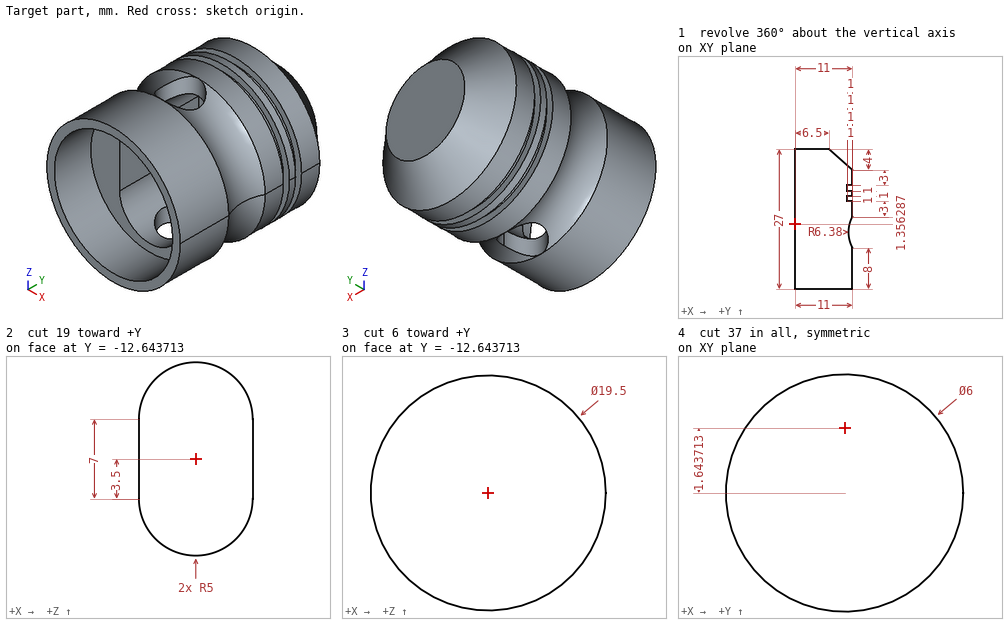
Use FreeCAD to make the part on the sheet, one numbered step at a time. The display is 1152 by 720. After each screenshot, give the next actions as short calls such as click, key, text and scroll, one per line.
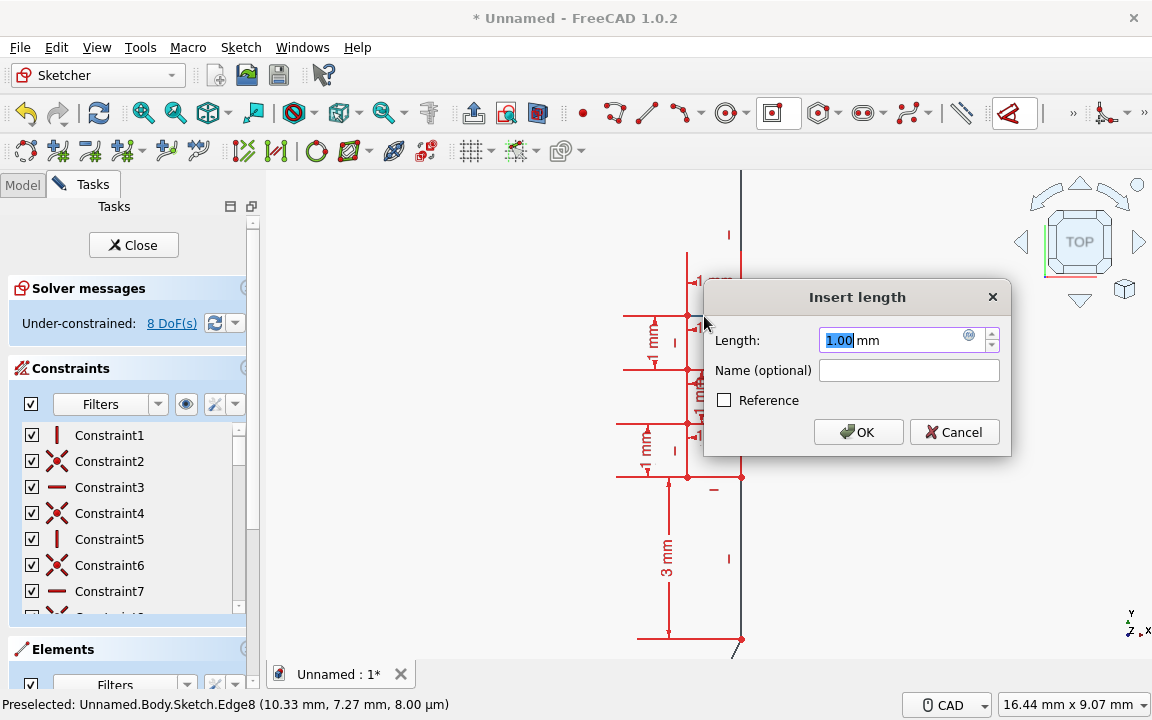
text(1)
key(Return)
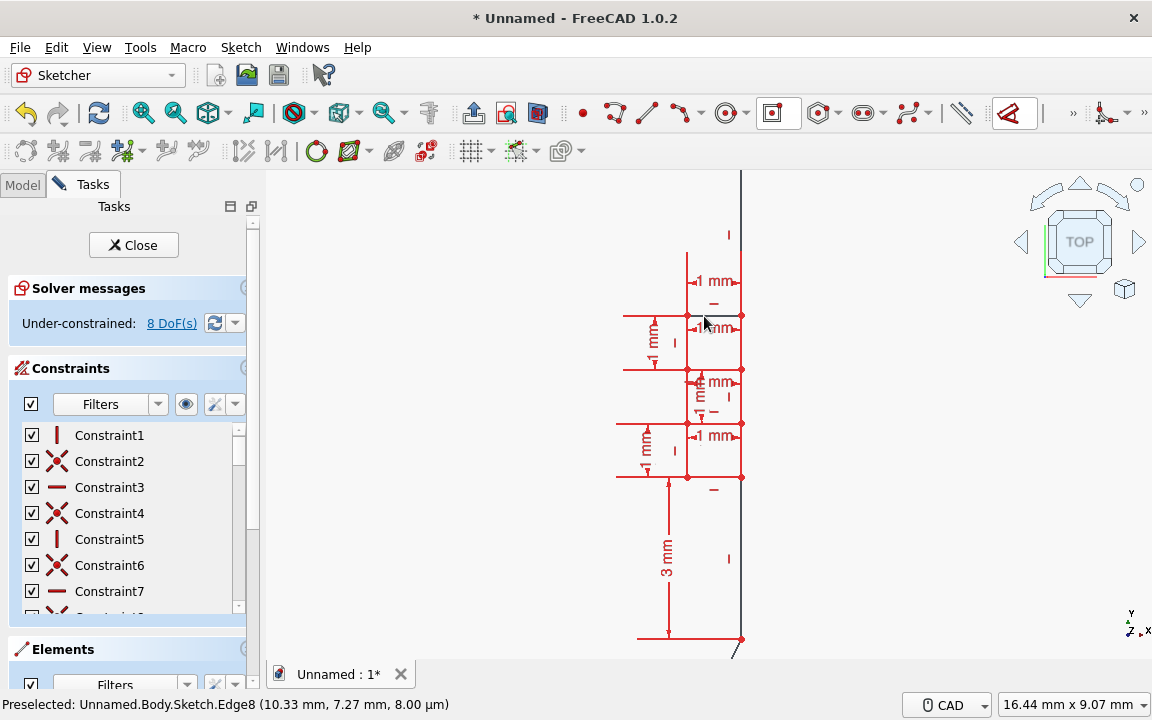
scroll(690, 352, down, 8)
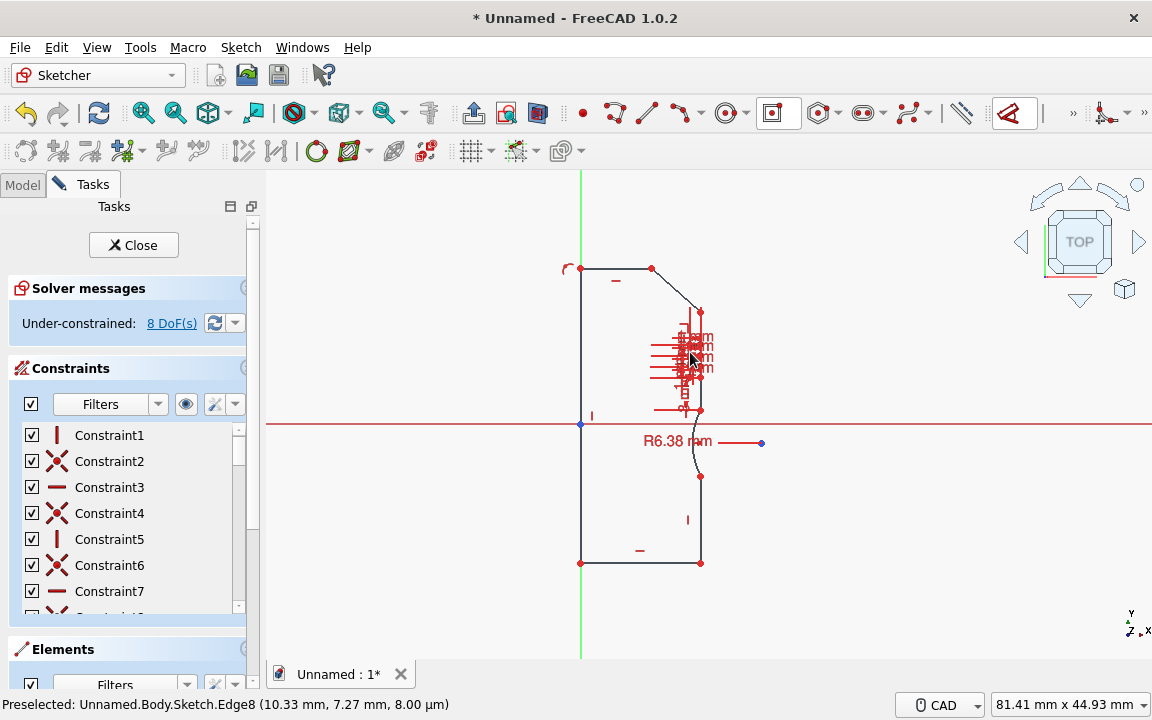
scroll(701, 335, up, 2)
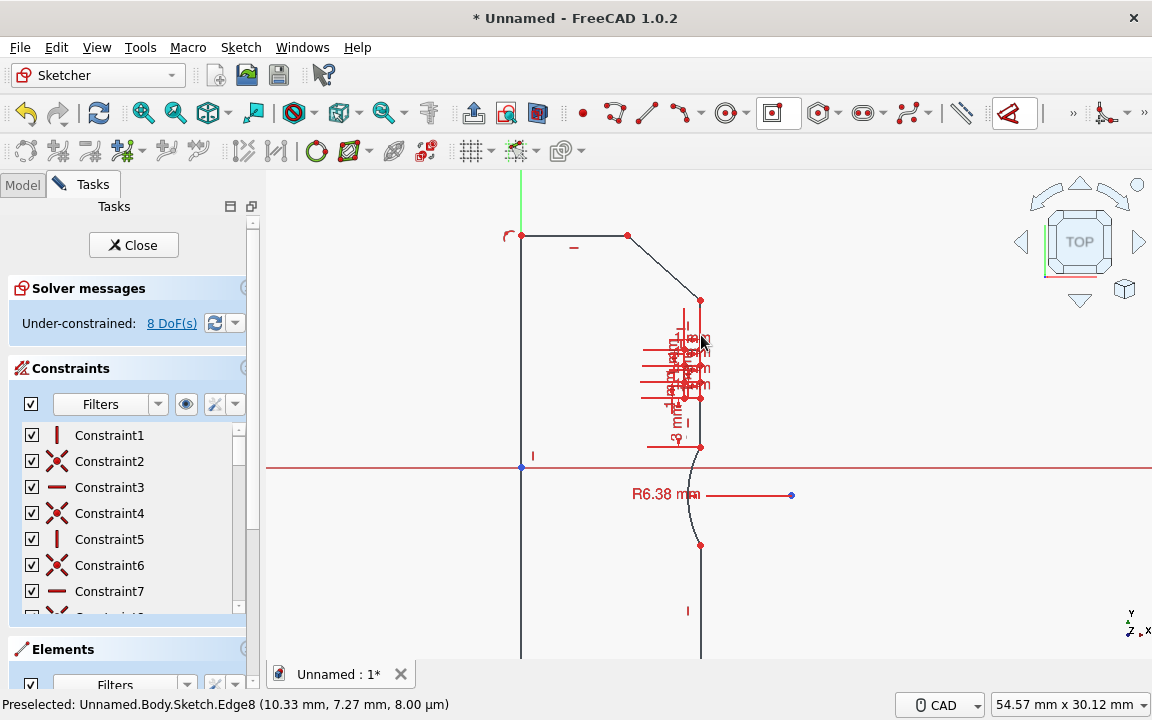
click(700, 315)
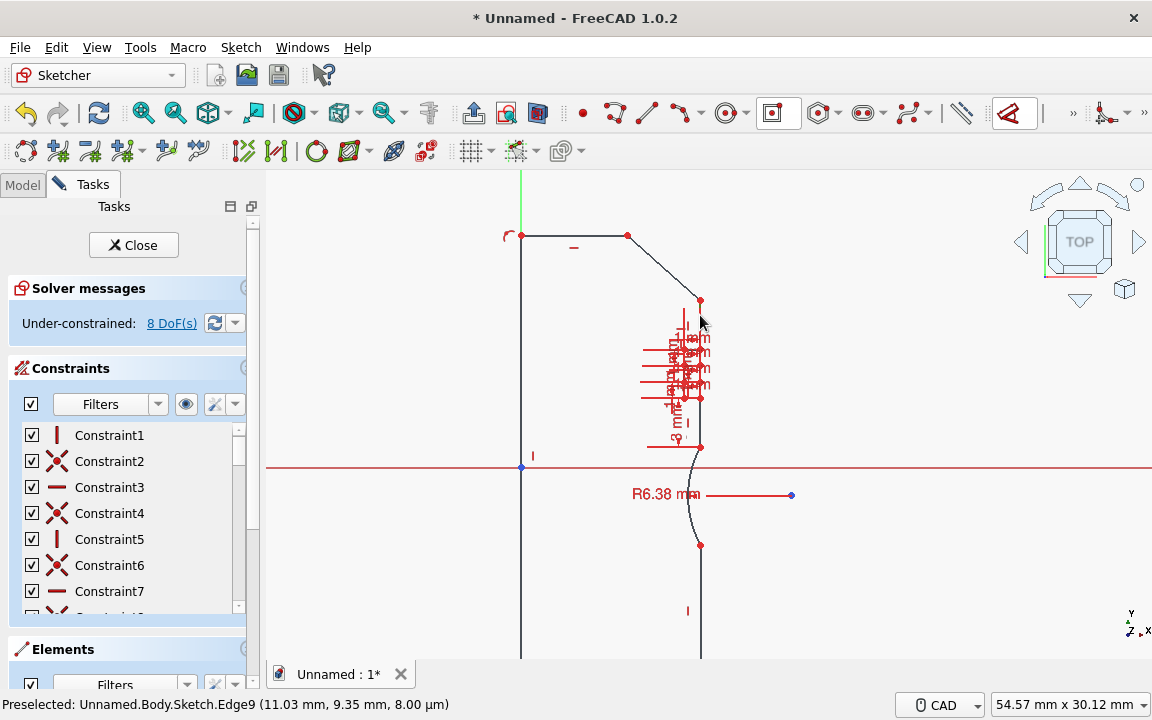
key(i)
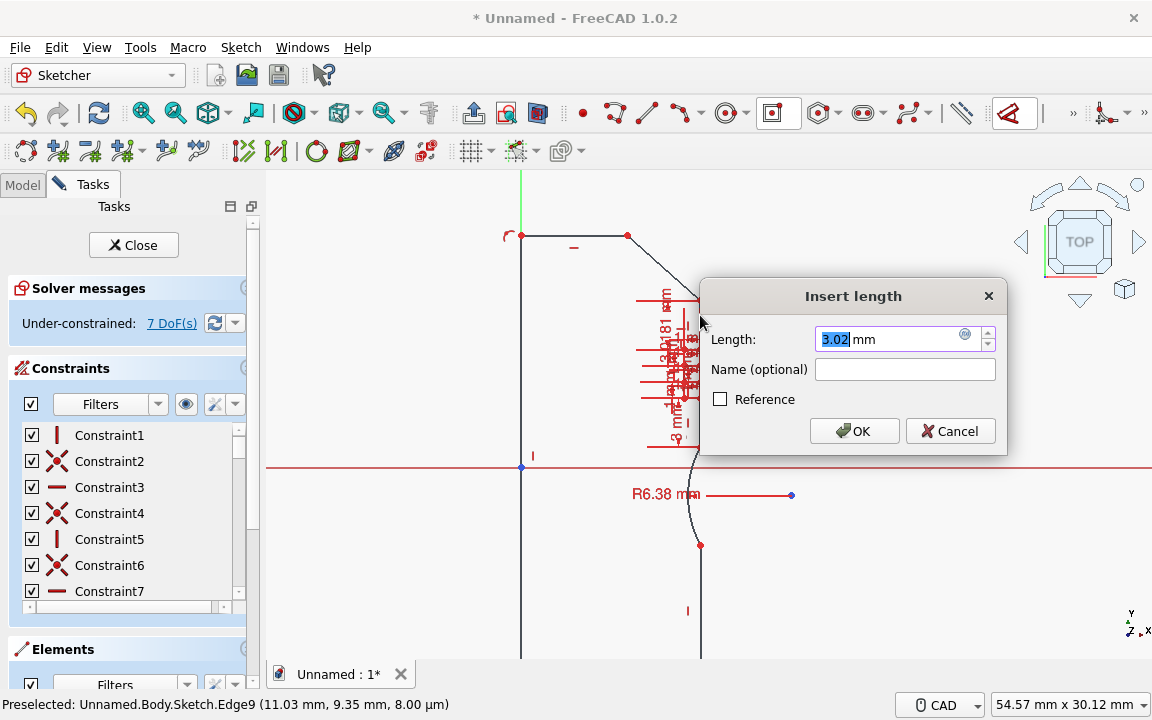
text(3)
key(Return)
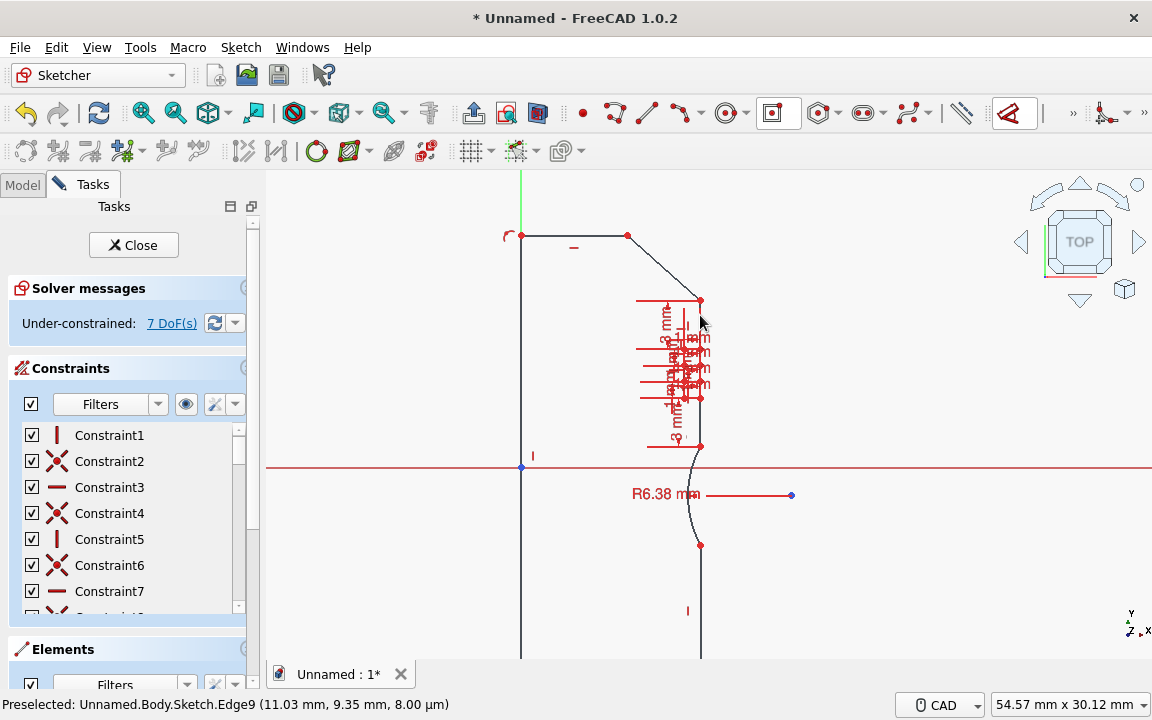
click(701, 584)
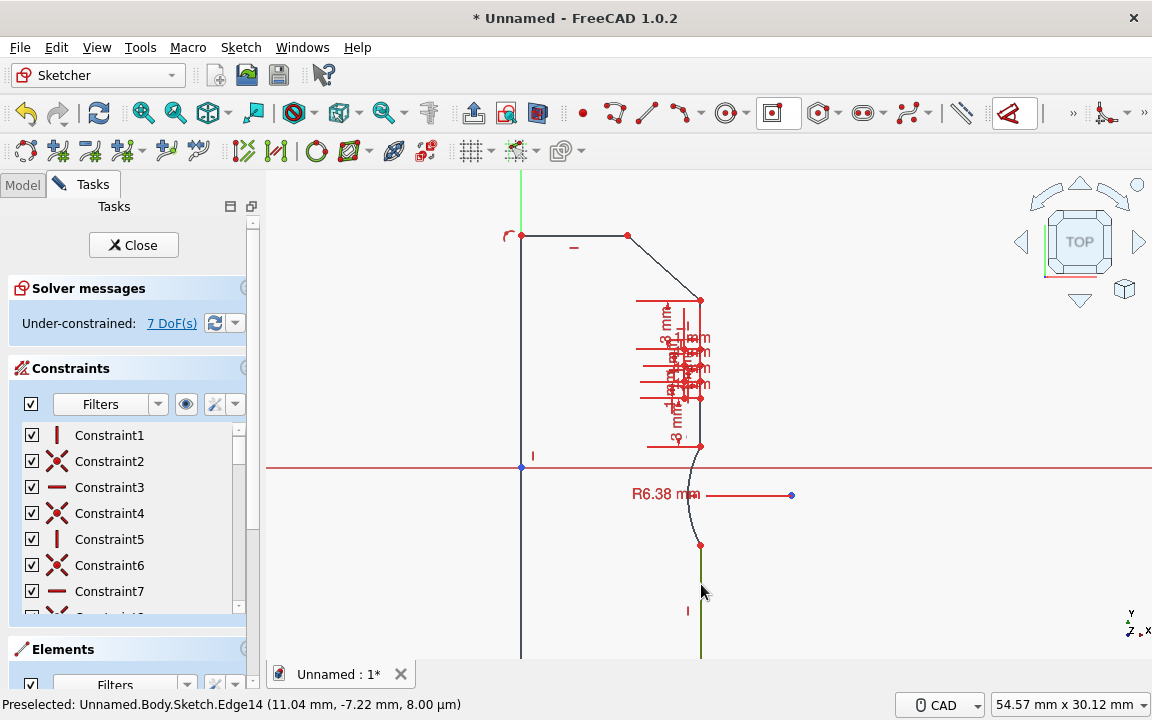
click(1032, 114)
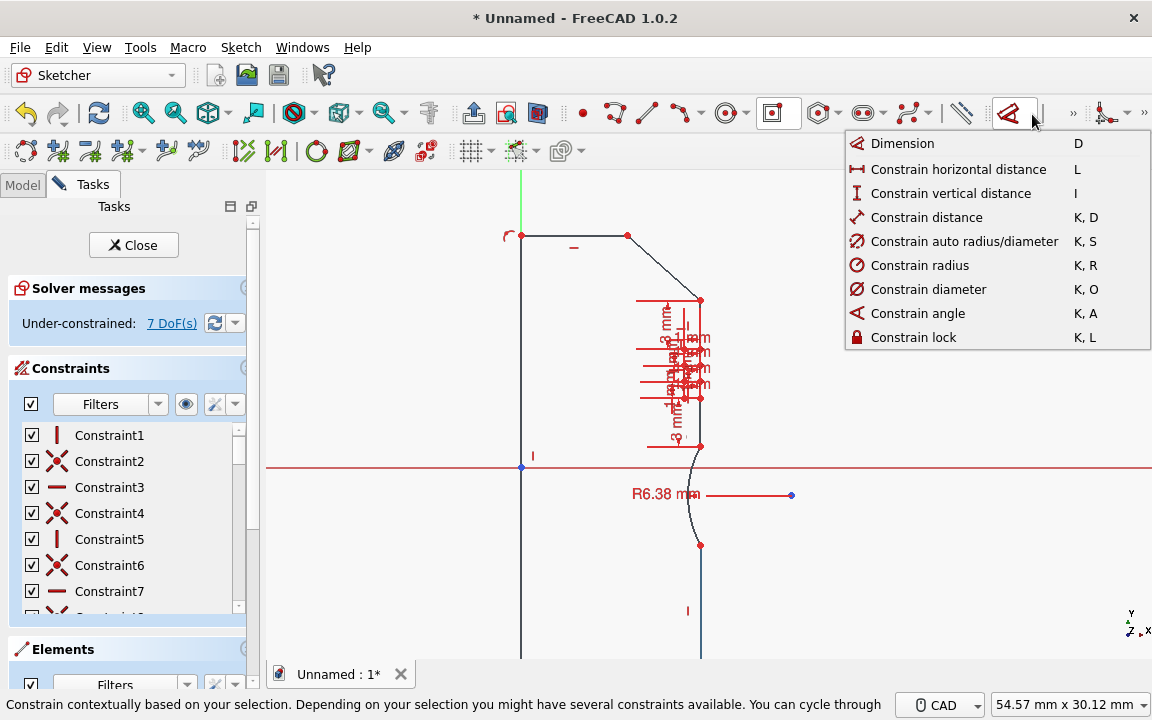
click(998, 193)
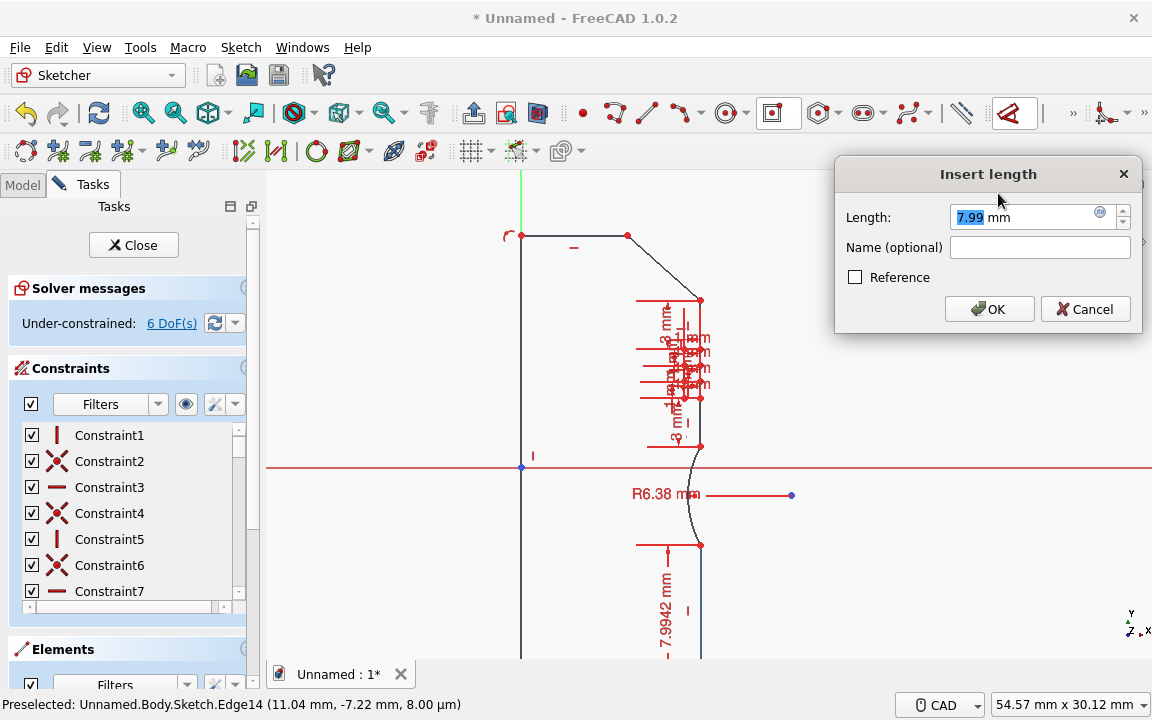
text(8)
key(Return)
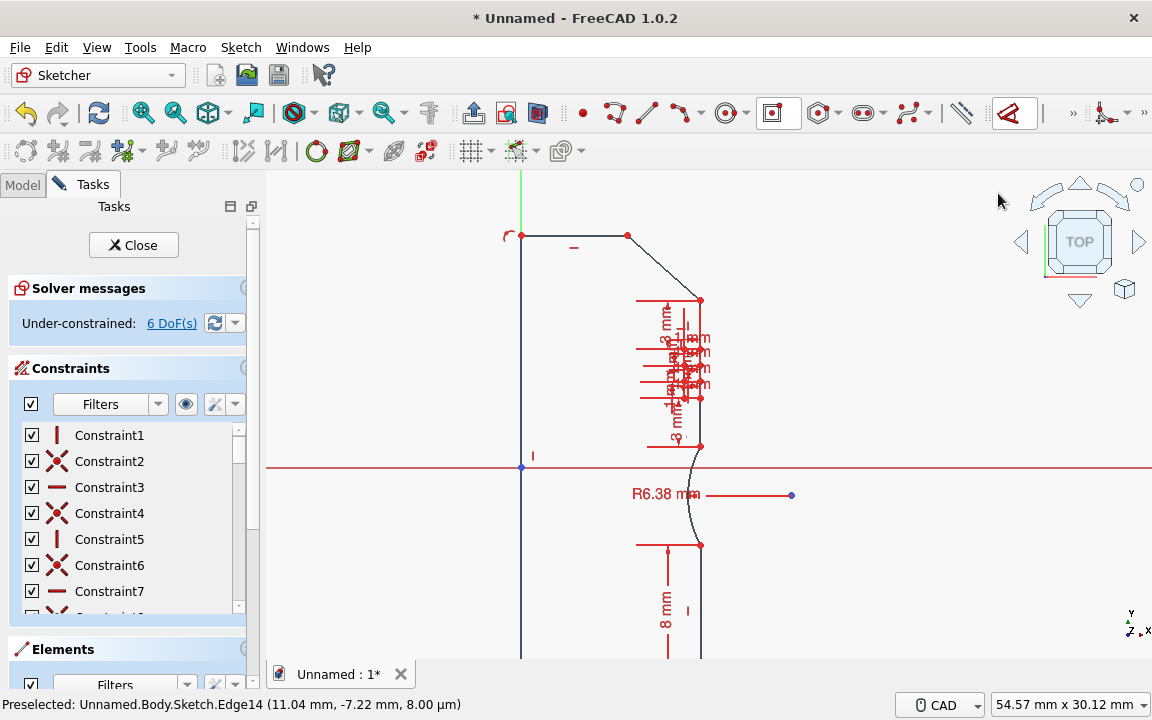
click(521, 367)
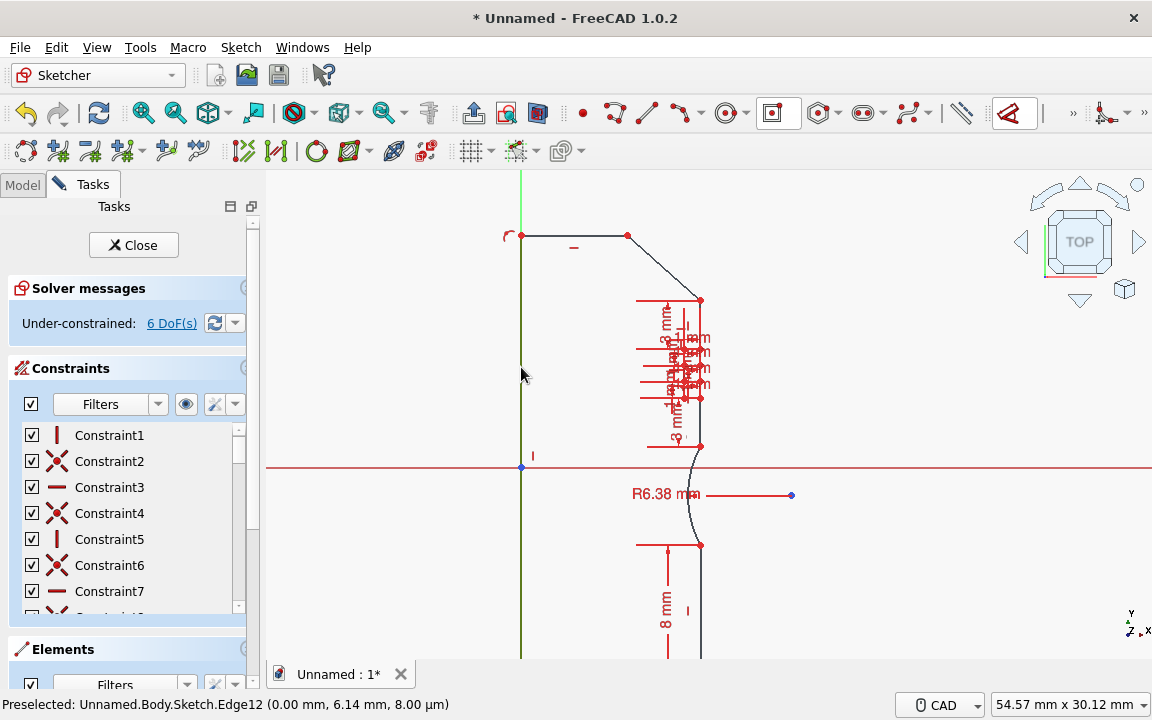
key(i)